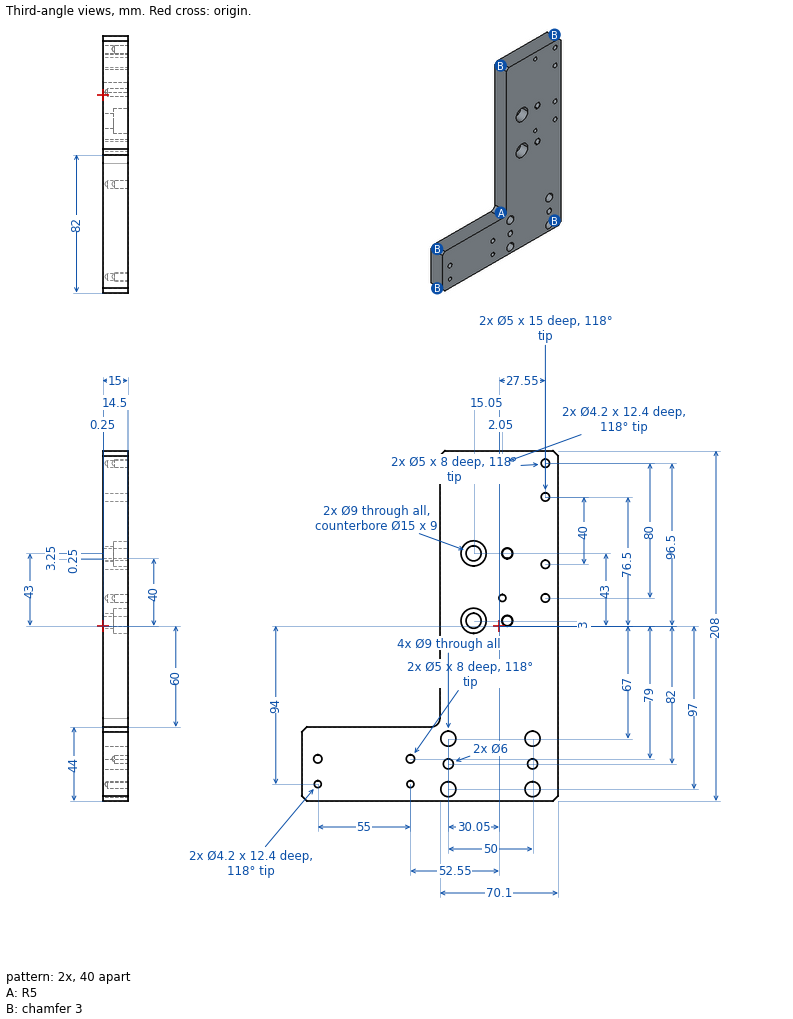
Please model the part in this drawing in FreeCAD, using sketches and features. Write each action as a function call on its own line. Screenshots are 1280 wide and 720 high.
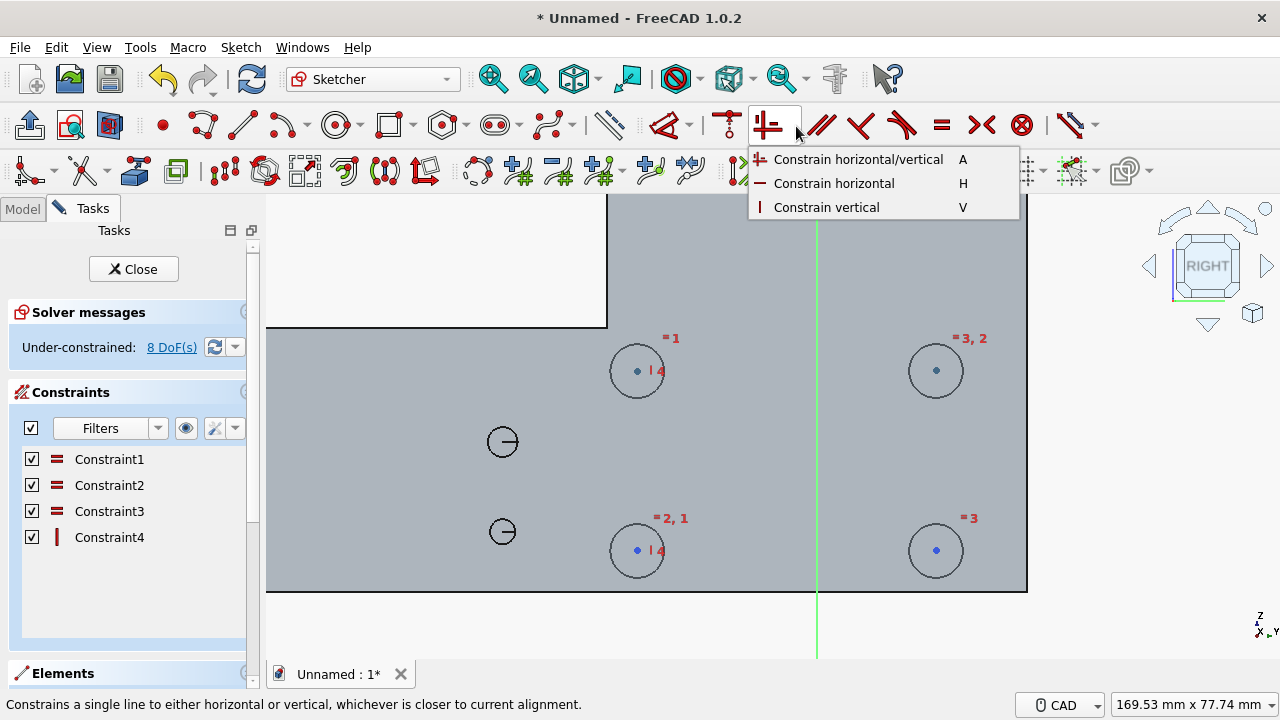
click(884, 183)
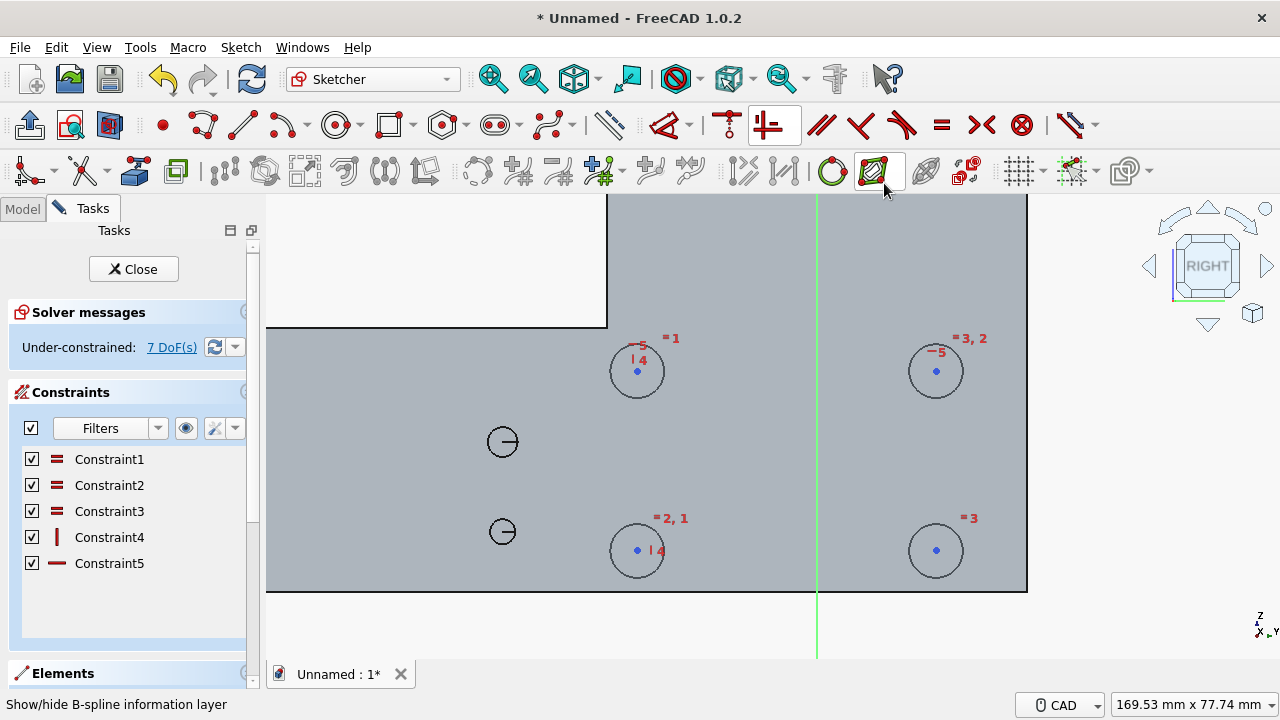
click(936, 371)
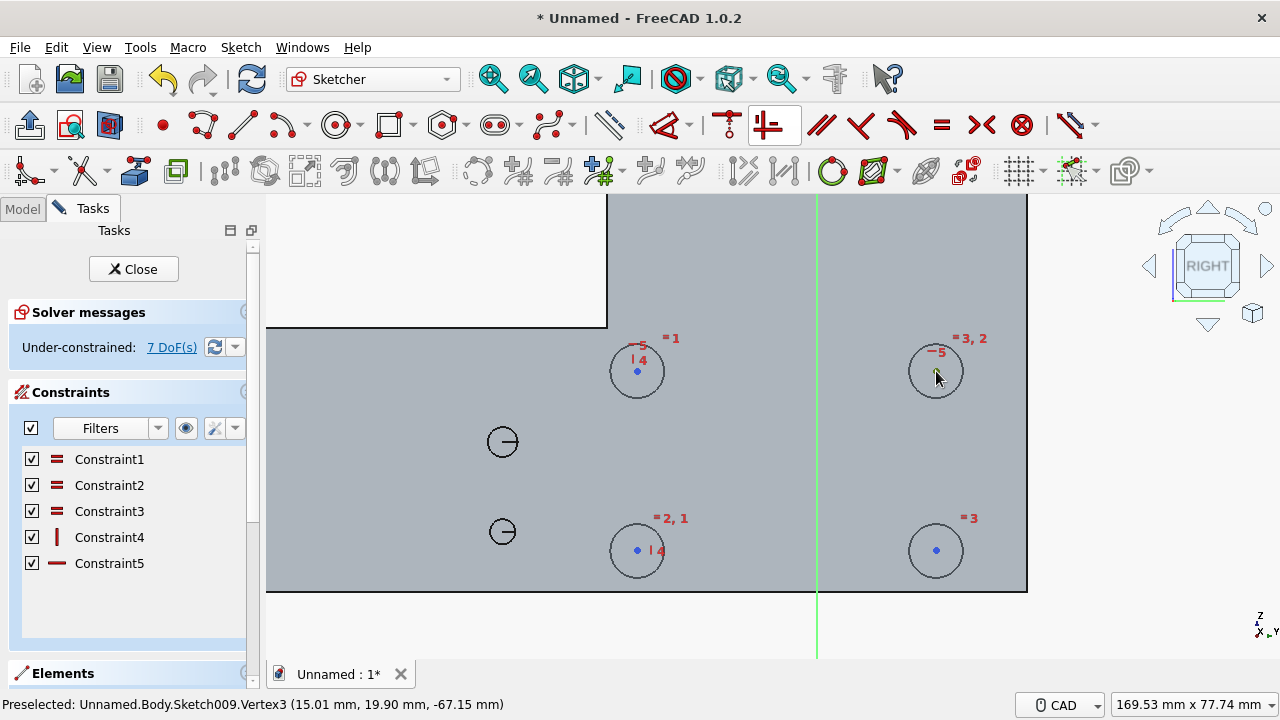
click(936, 551)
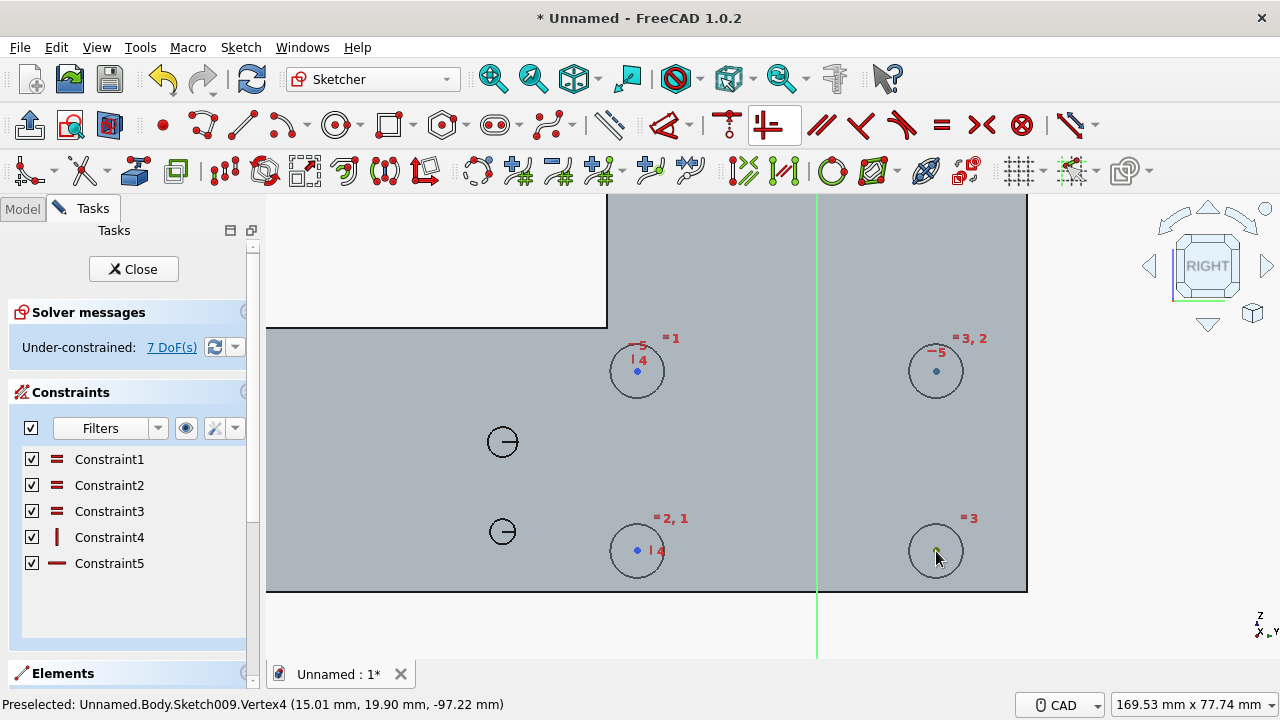
key(v)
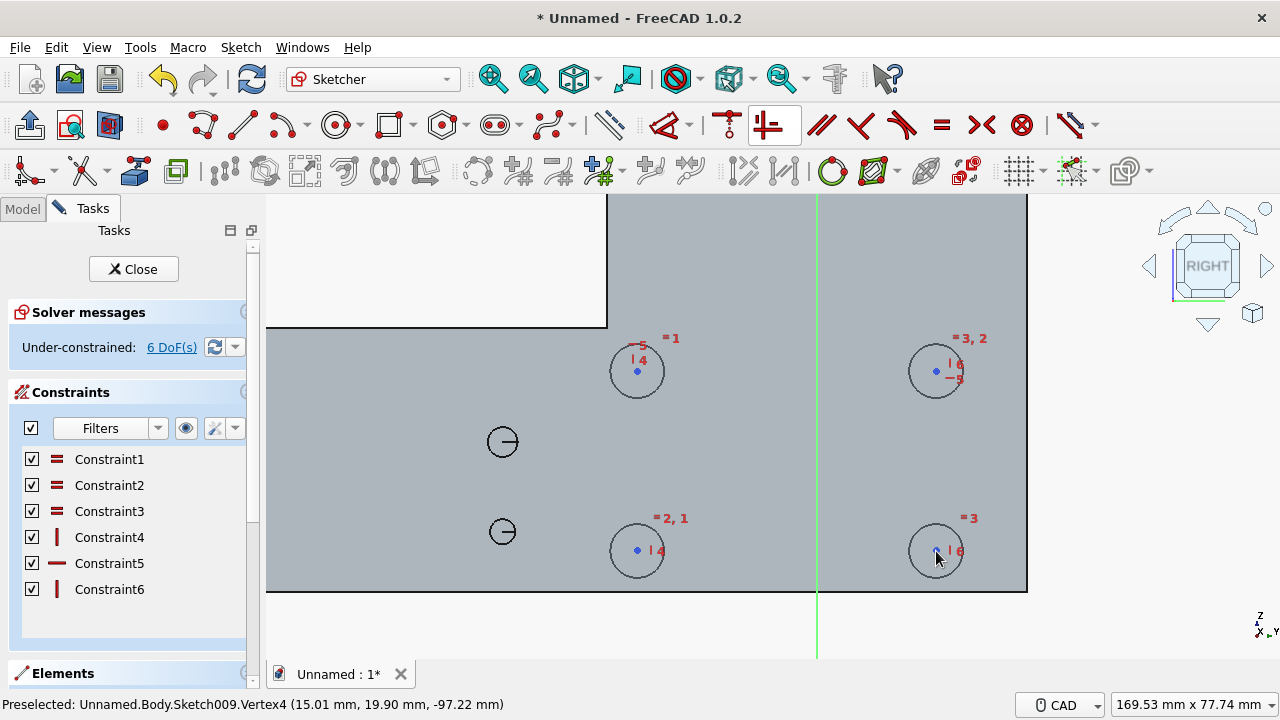
click(637, 551)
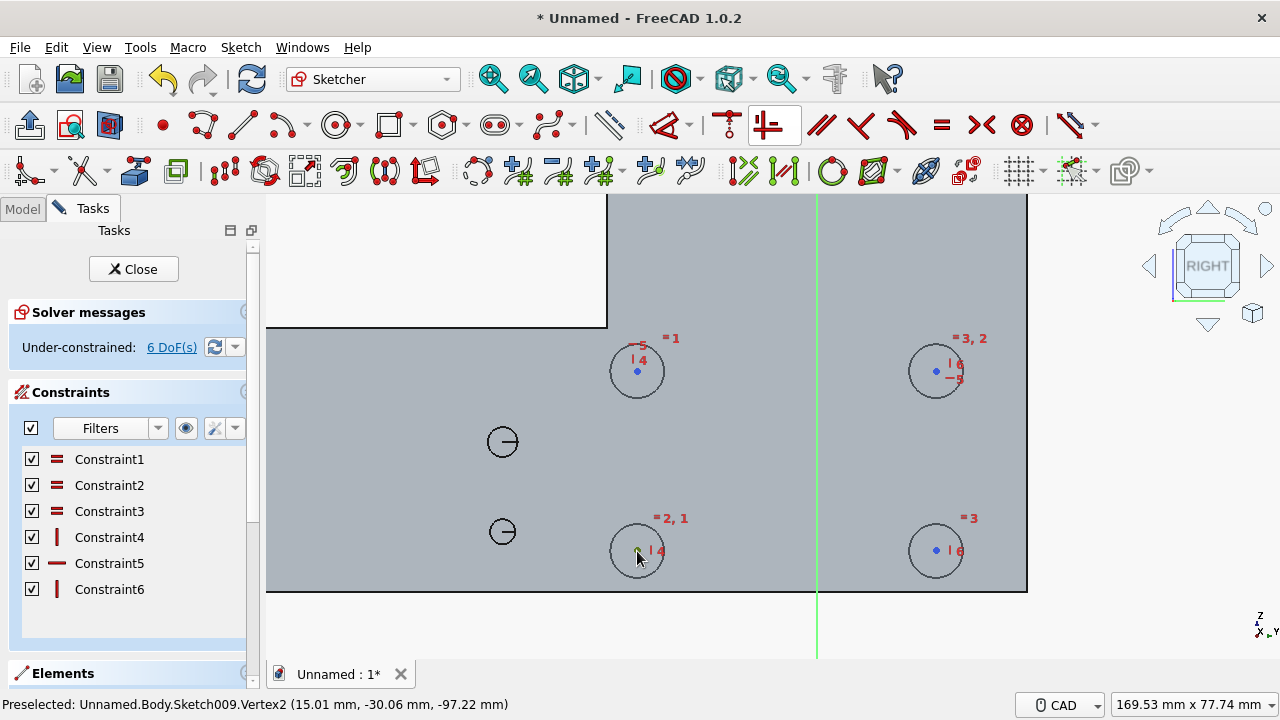
click(936, 551)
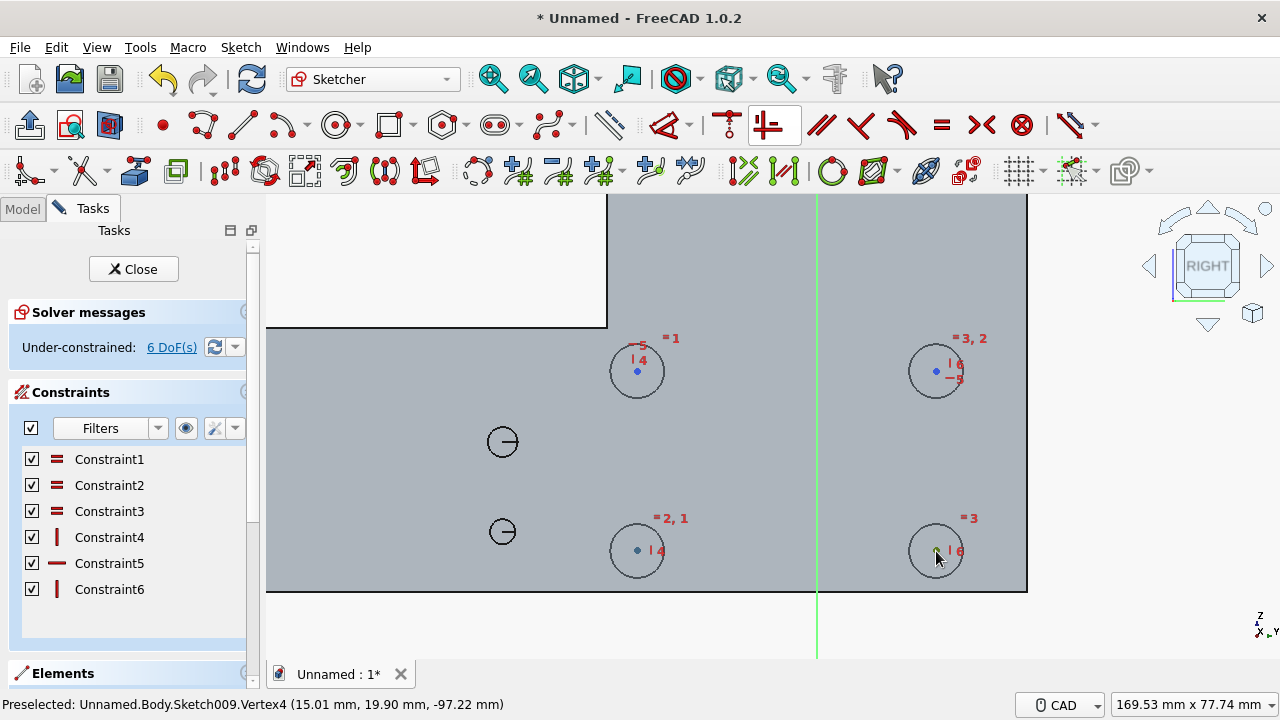
key(h)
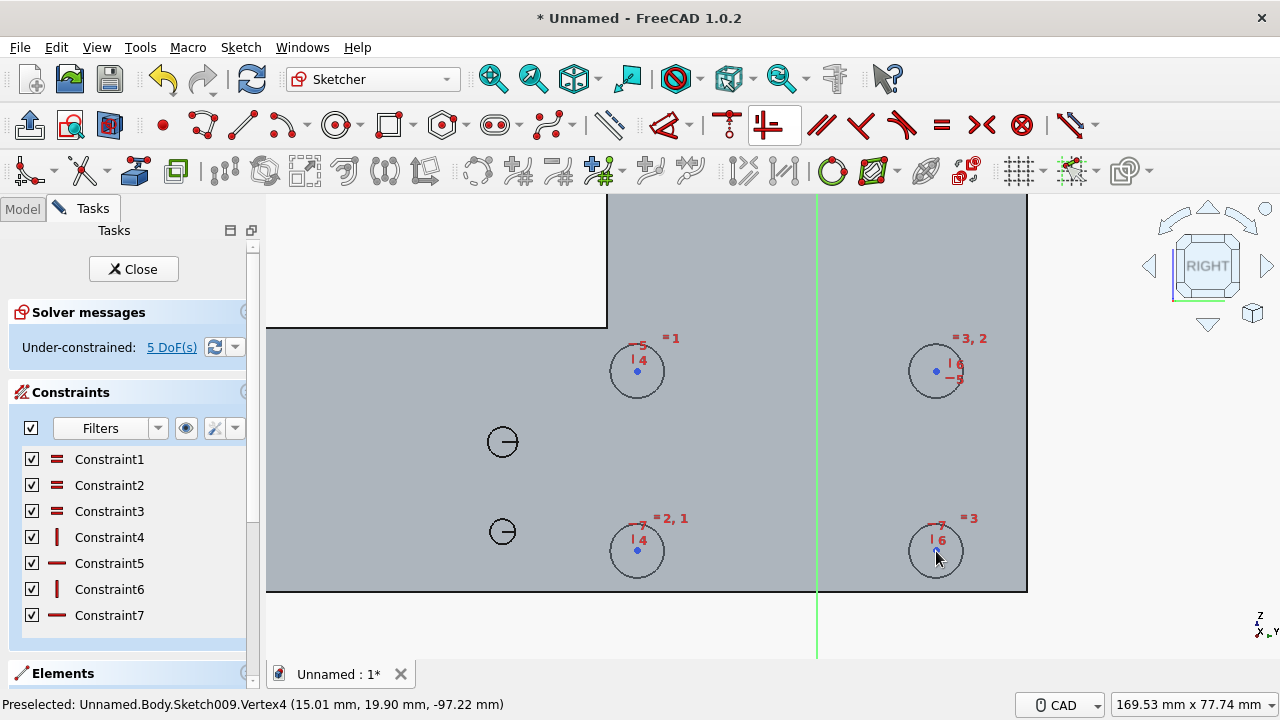
click(664, 126)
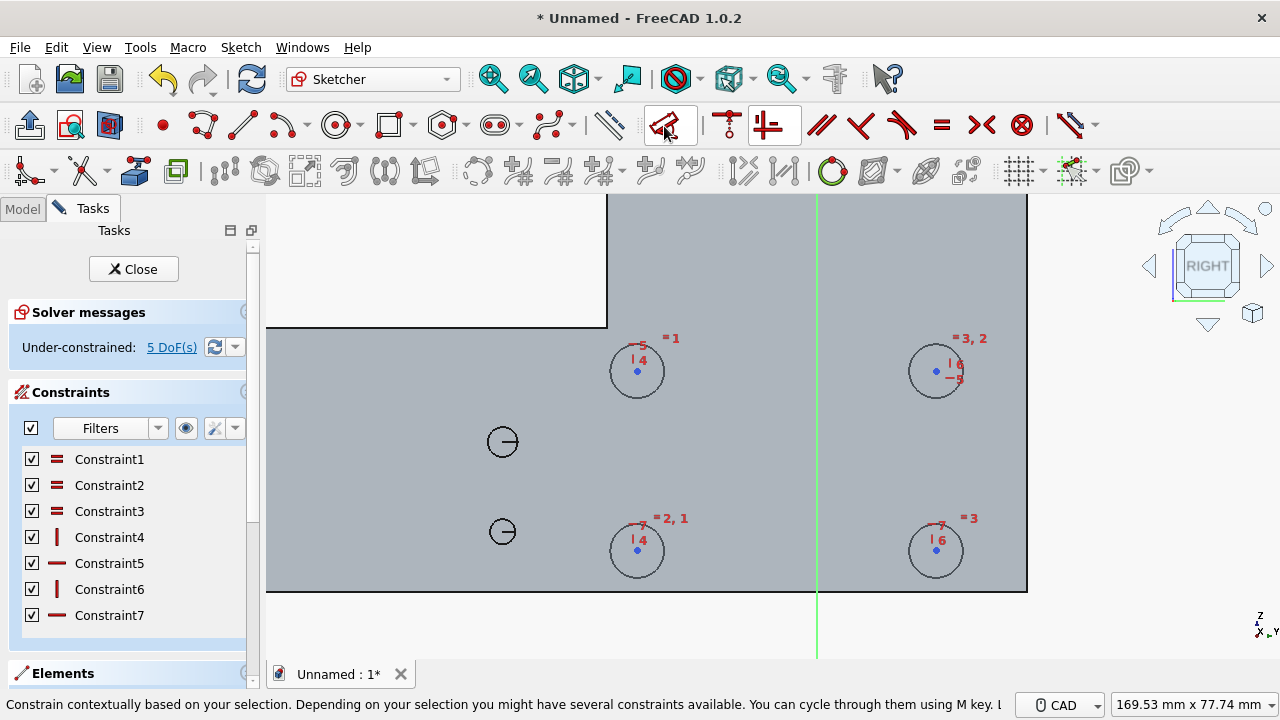
click(656, 352)
click(678, 329)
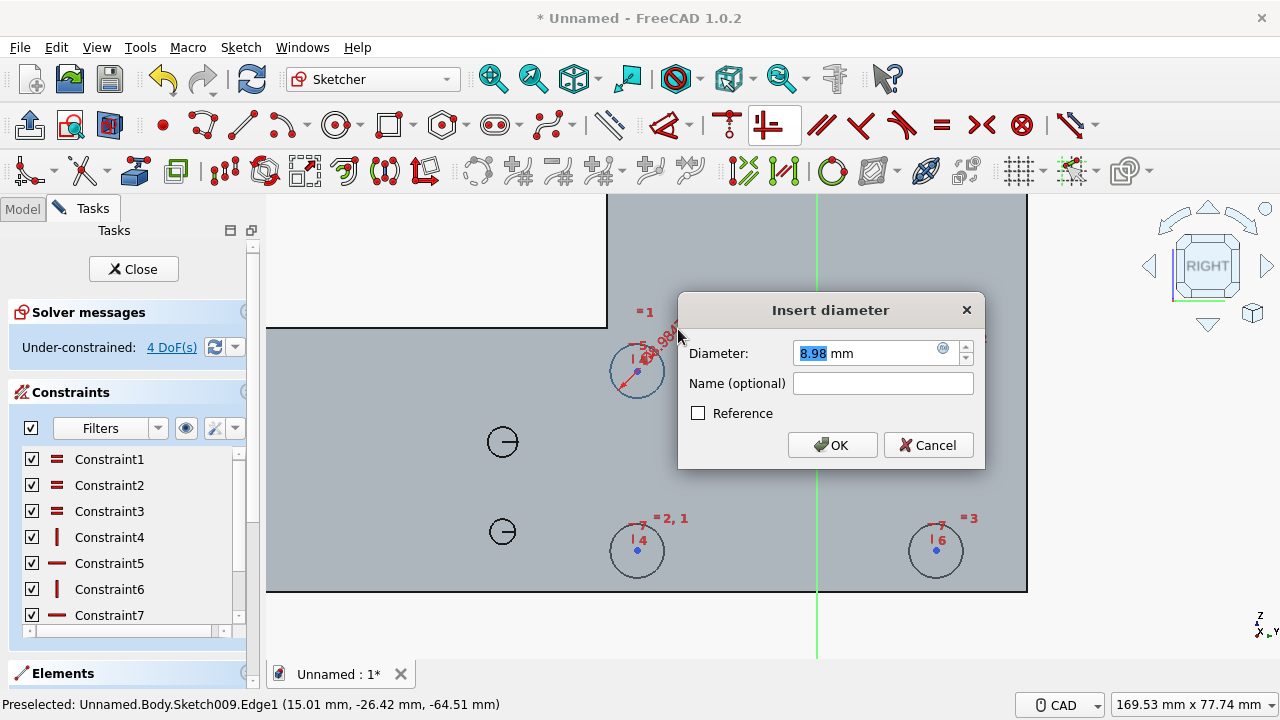
text(9)
key(Return)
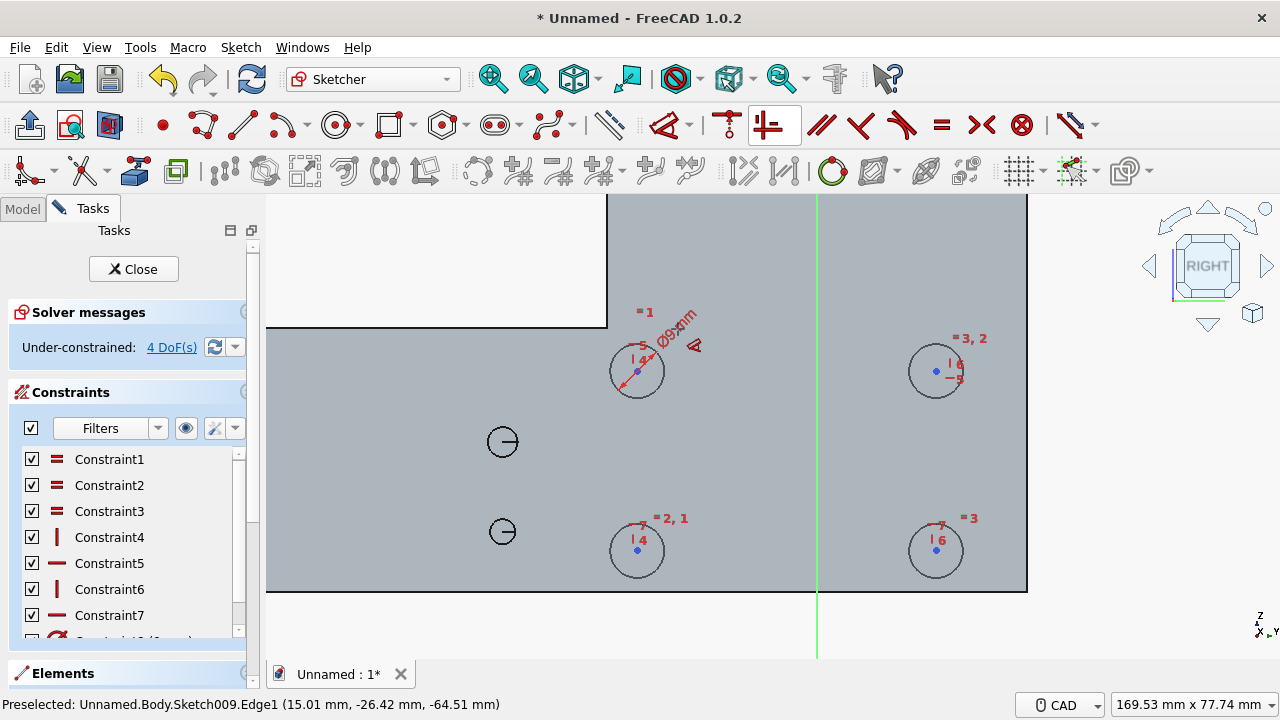
click(637, 371)
click(603, 297)